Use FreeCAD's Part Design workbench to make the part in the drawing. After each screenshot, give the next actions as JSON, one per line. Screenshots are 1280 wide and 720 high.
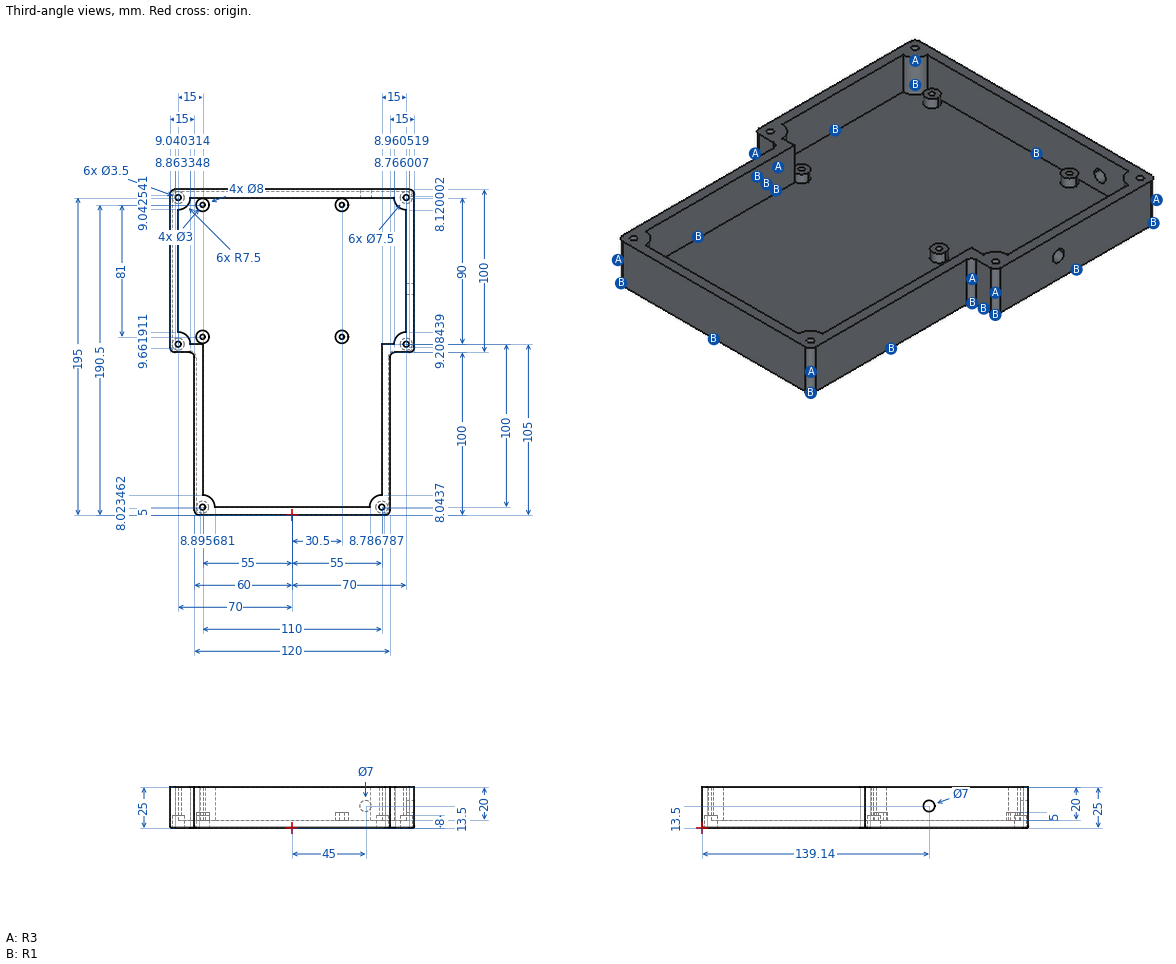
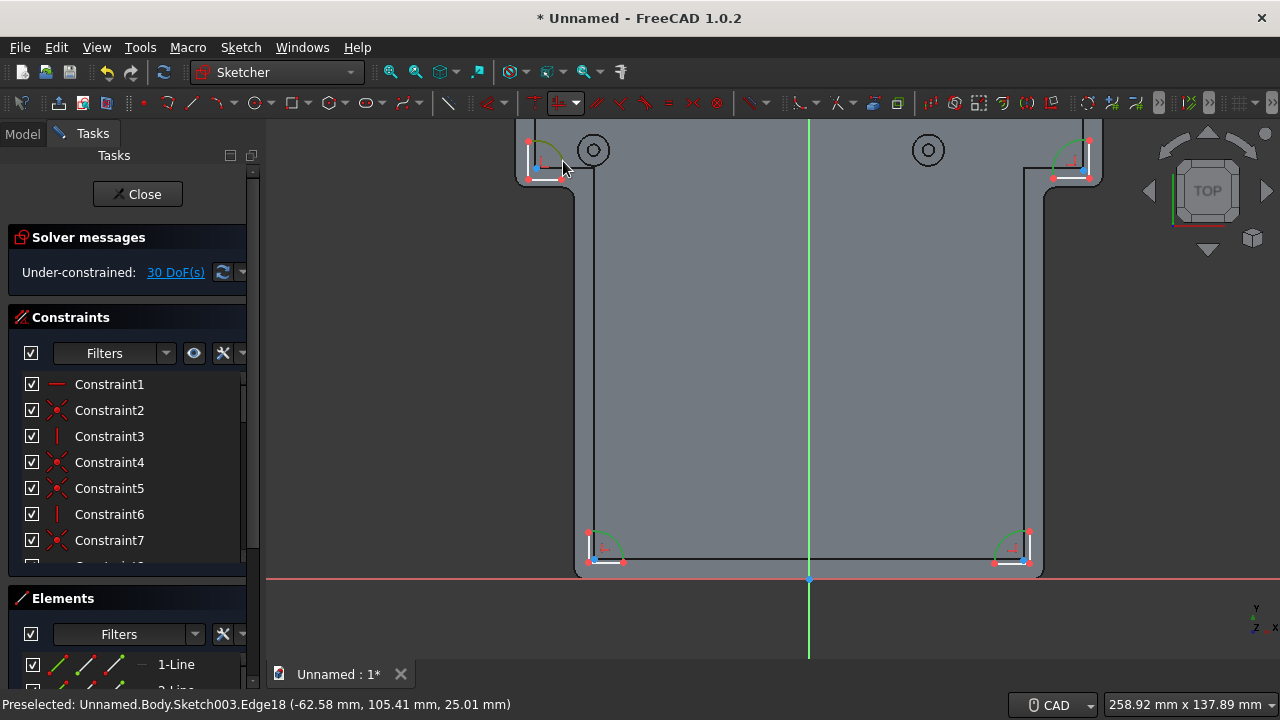
{"action": "key", "text": "e"}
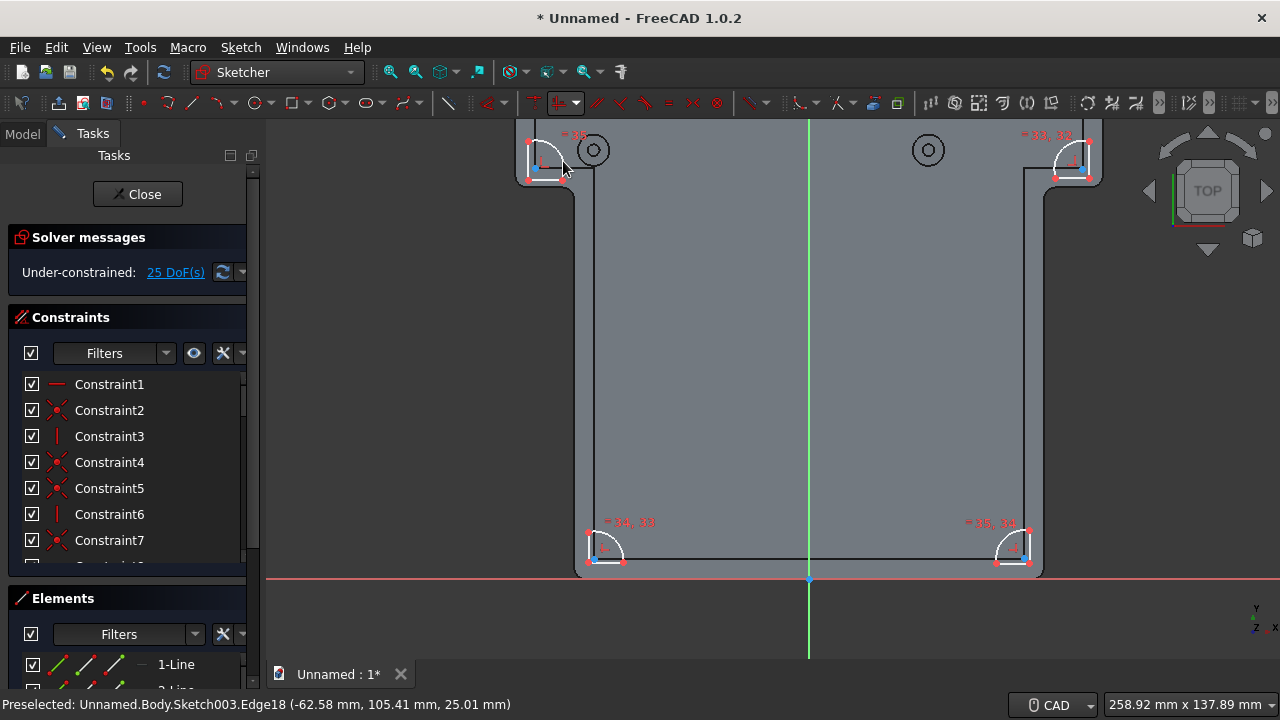
{"action": "left_click", "coordinate": [488, 104]}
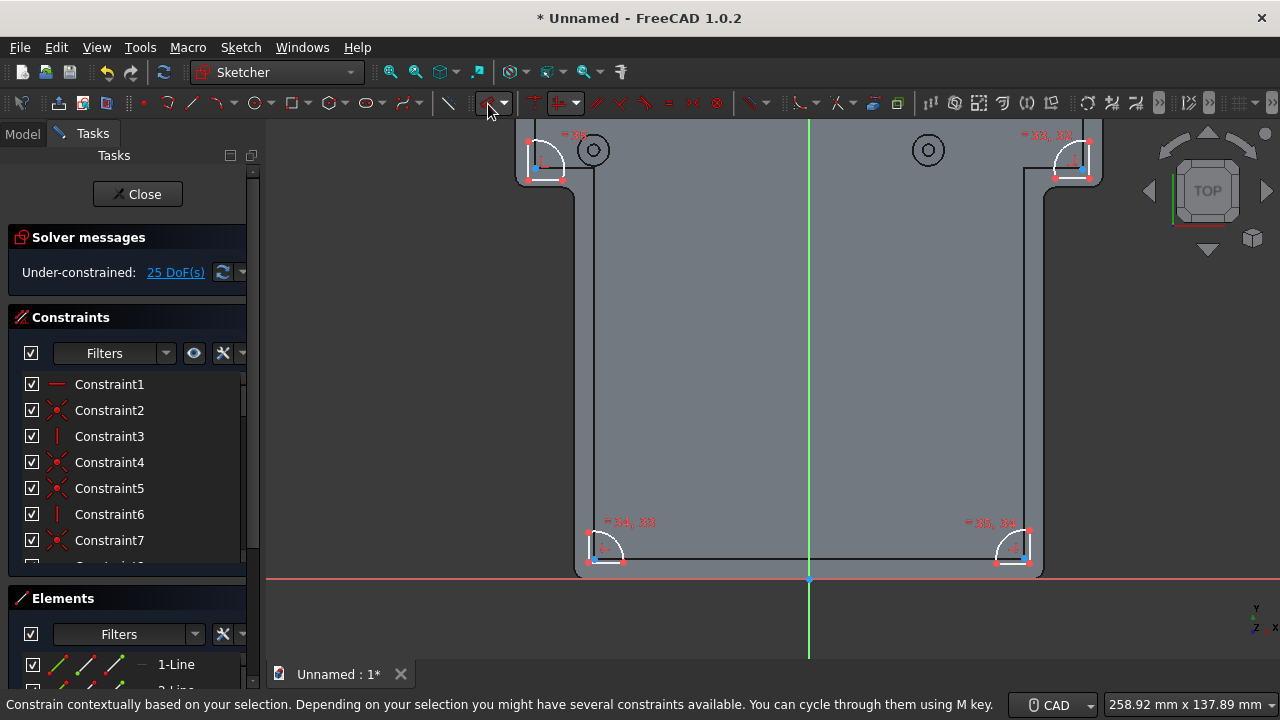
{"action": "scroll", "coordinate": [620, 548], "scroll_direction": "down", "scroll_amount": 4}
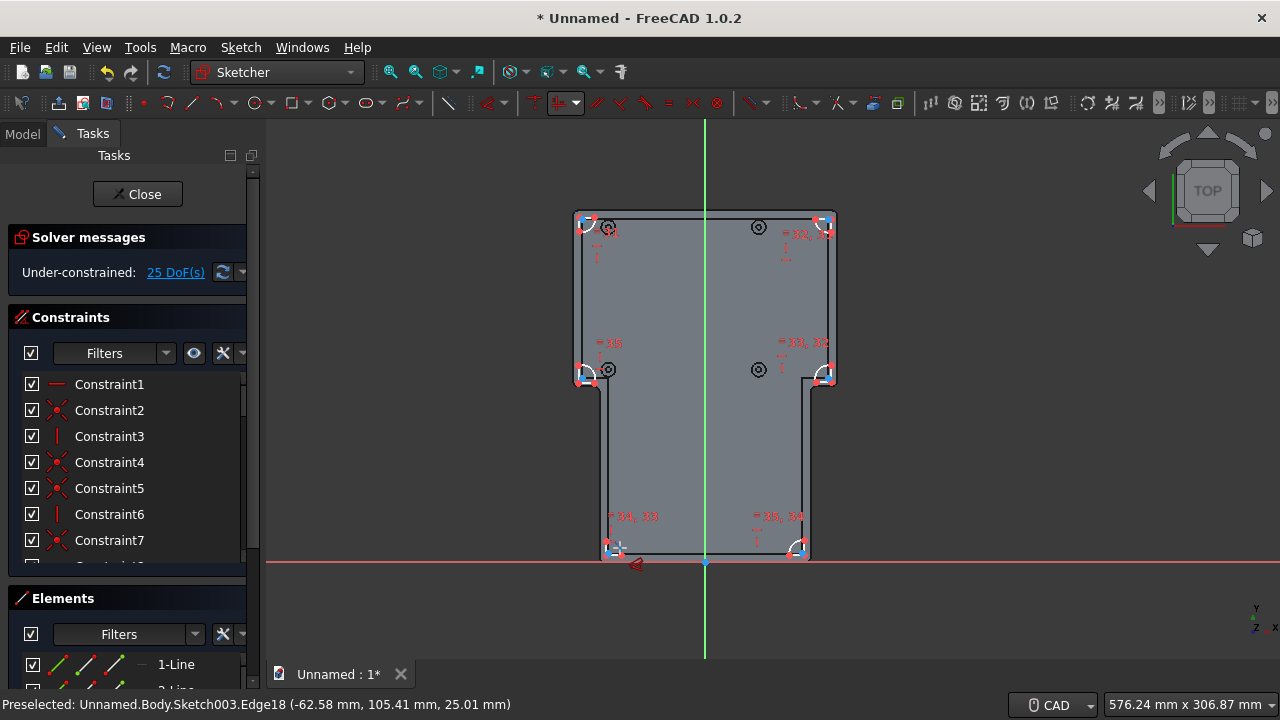
{"action": "scroll", "coordinate": [587, 231], "scroll_direction": "up", "scroll_amount": 6}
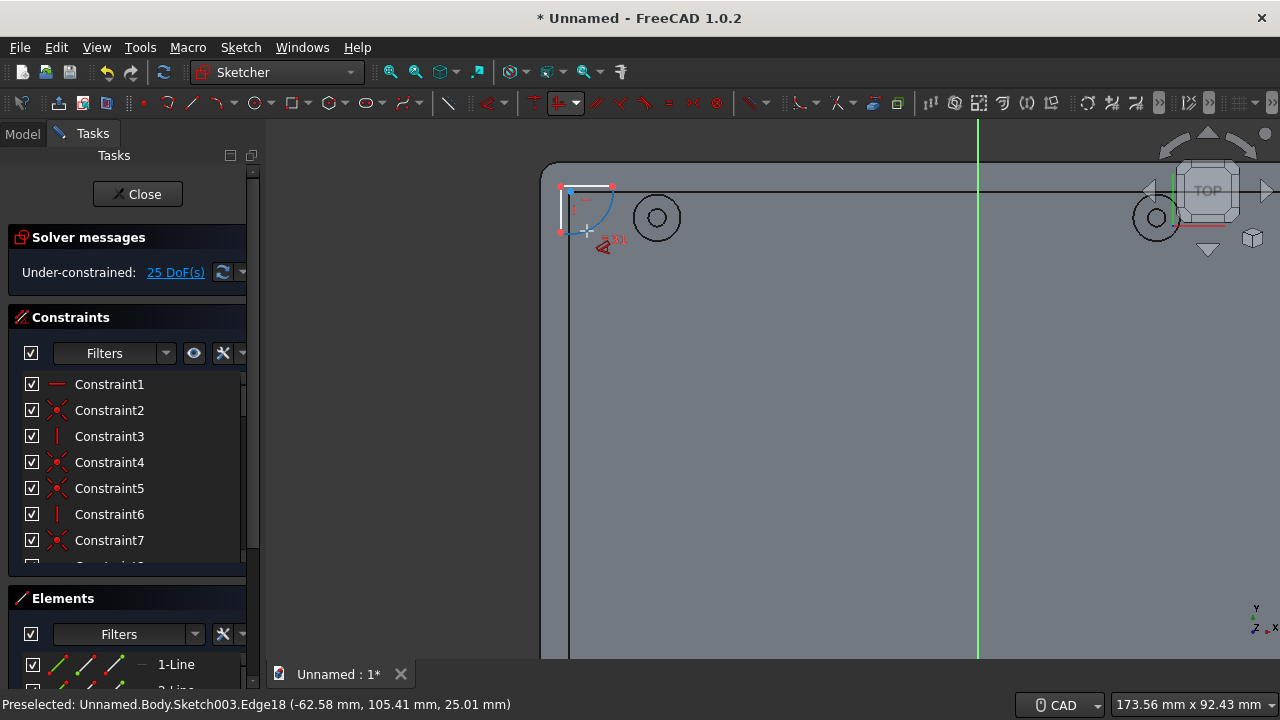
{"action": "left_click", "coordinate": [585, 232]}
{"action": "left_click", "coordinate": [596, 262]}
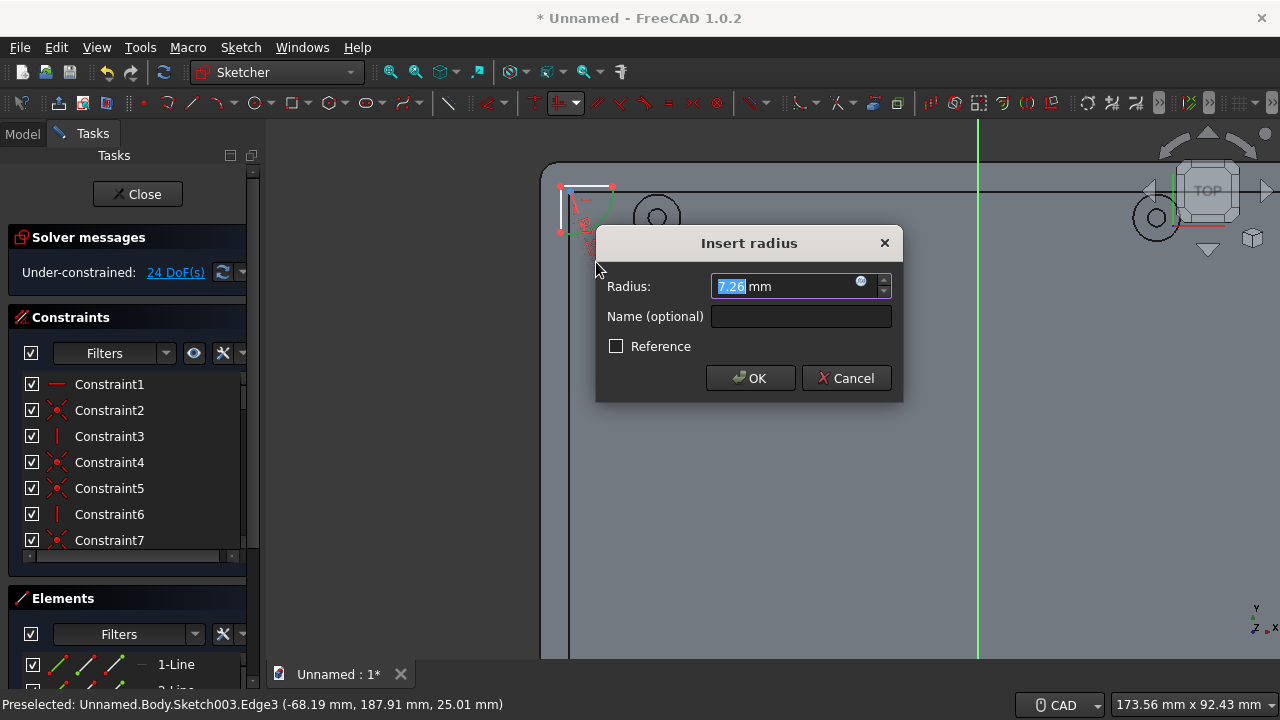
{"action": "type", "text": "7.5"}
{"action": "key", "text": "Return"}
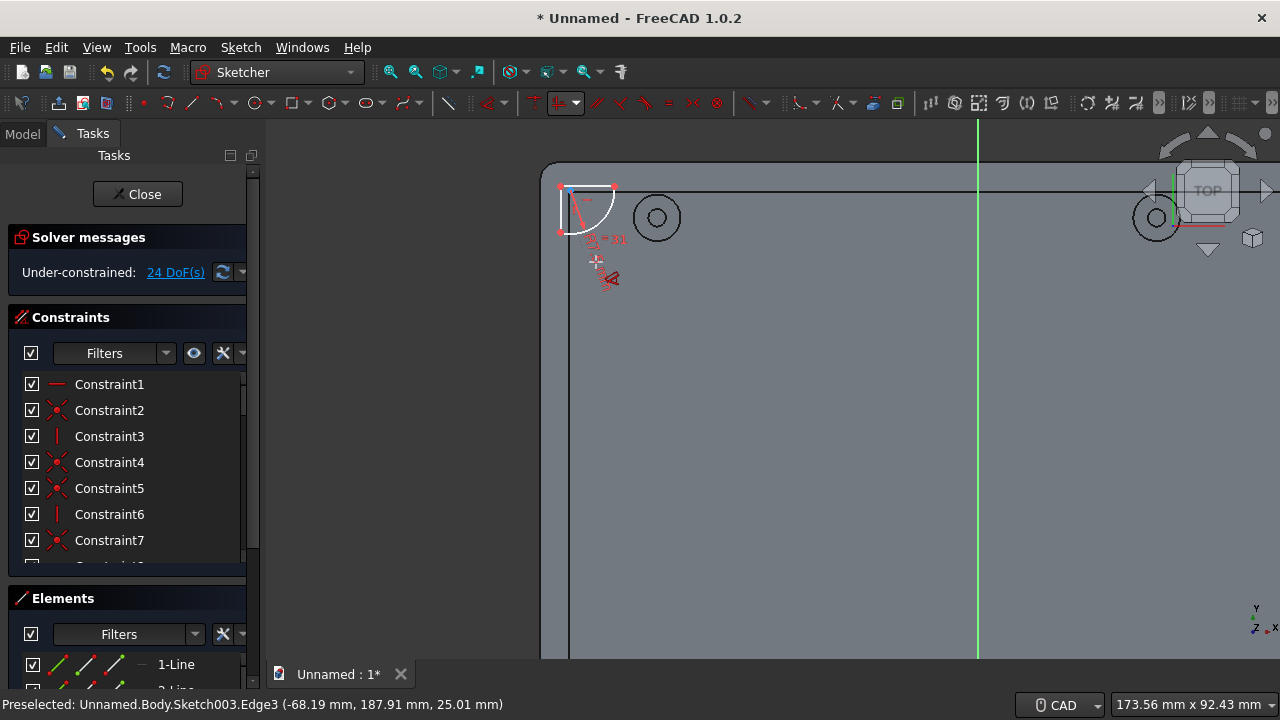
{"action": "scroll", "coordinate": [587, 231], "scroll_direction": "down", "scroll_amount": 6}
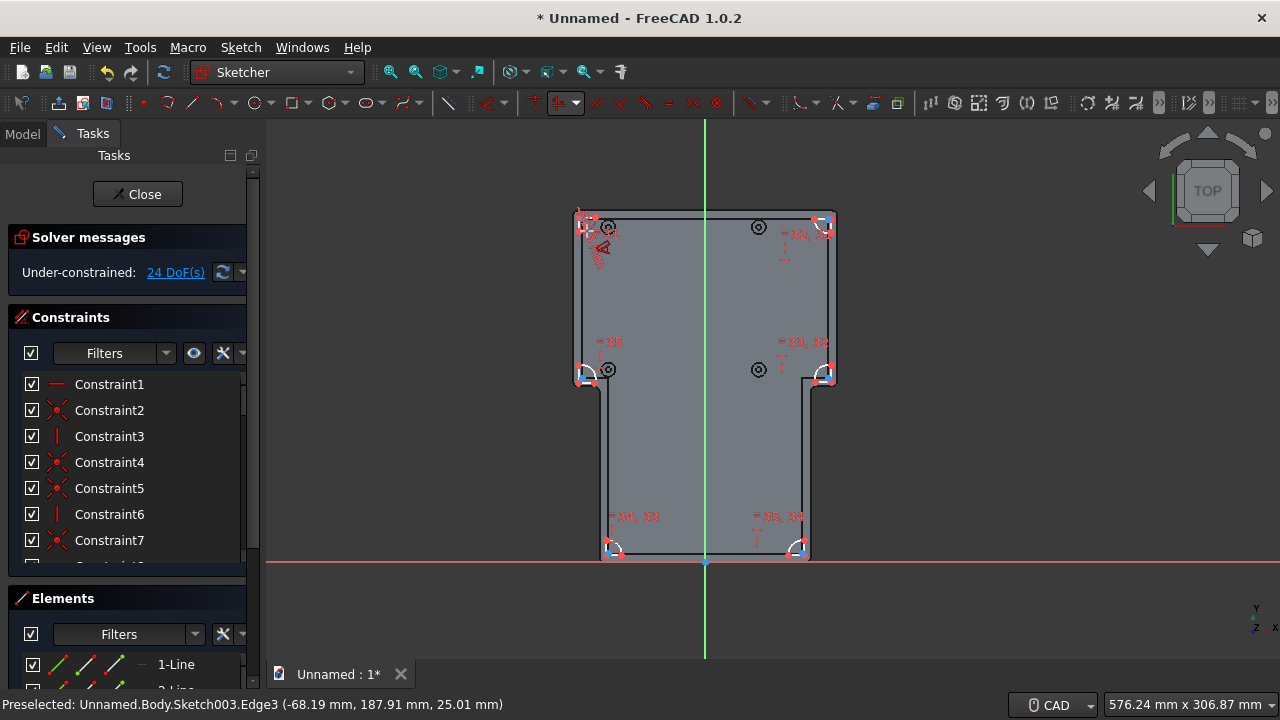
{"action": "scroll", "coordinate": [608, 554], "scroll_direction": "up", "scroll_amount": 8}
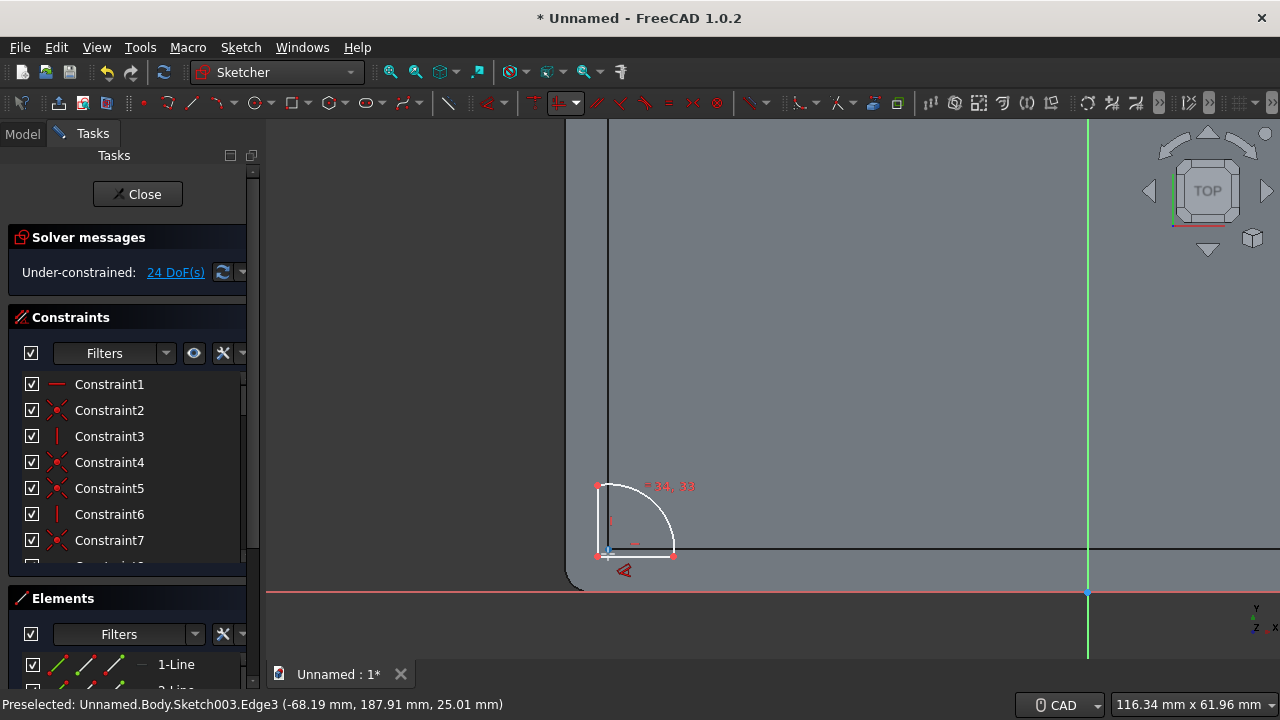
{"action": "left_click", "coordinate": [609, 550]}
{"action": "left_click", "coordinate": [575, 571]}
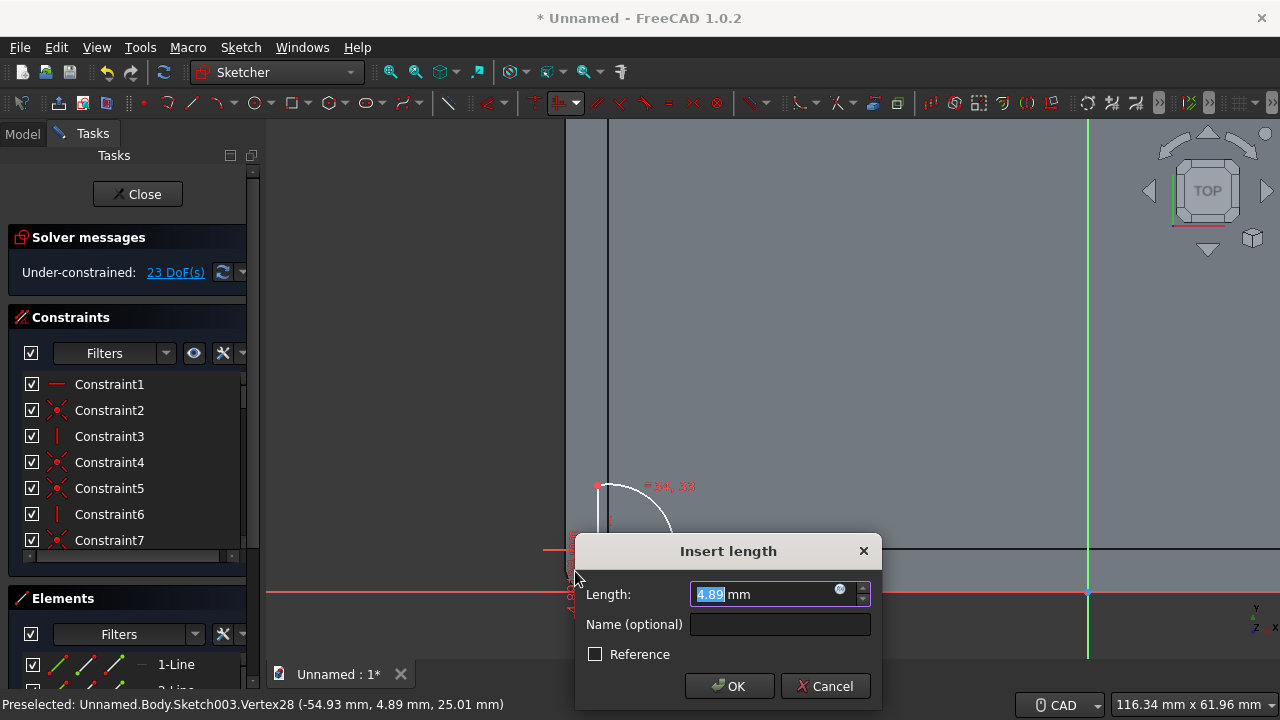
{"action": "type", "text": "5"}
{"action": "key", "text": "Return"}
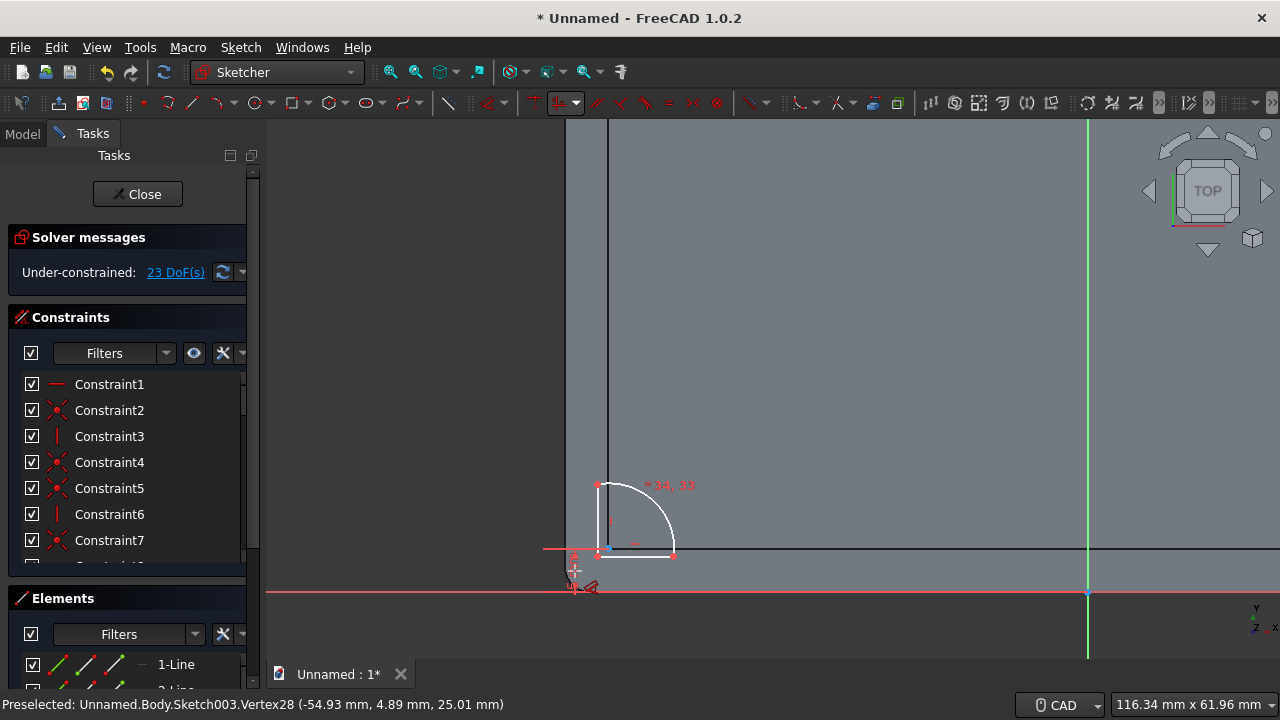
{"action": "scroll", "coordinate": [608, 554], "scroll_direction": "down", "scroll_amount": 8}